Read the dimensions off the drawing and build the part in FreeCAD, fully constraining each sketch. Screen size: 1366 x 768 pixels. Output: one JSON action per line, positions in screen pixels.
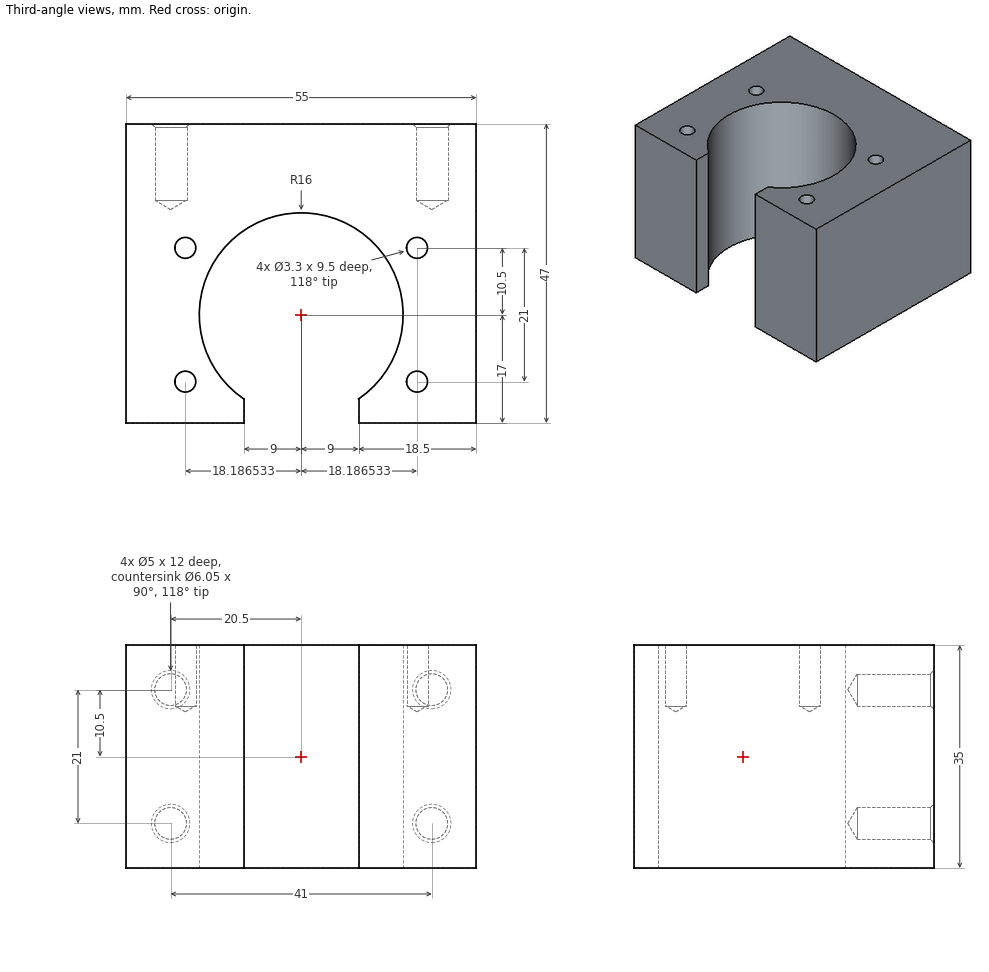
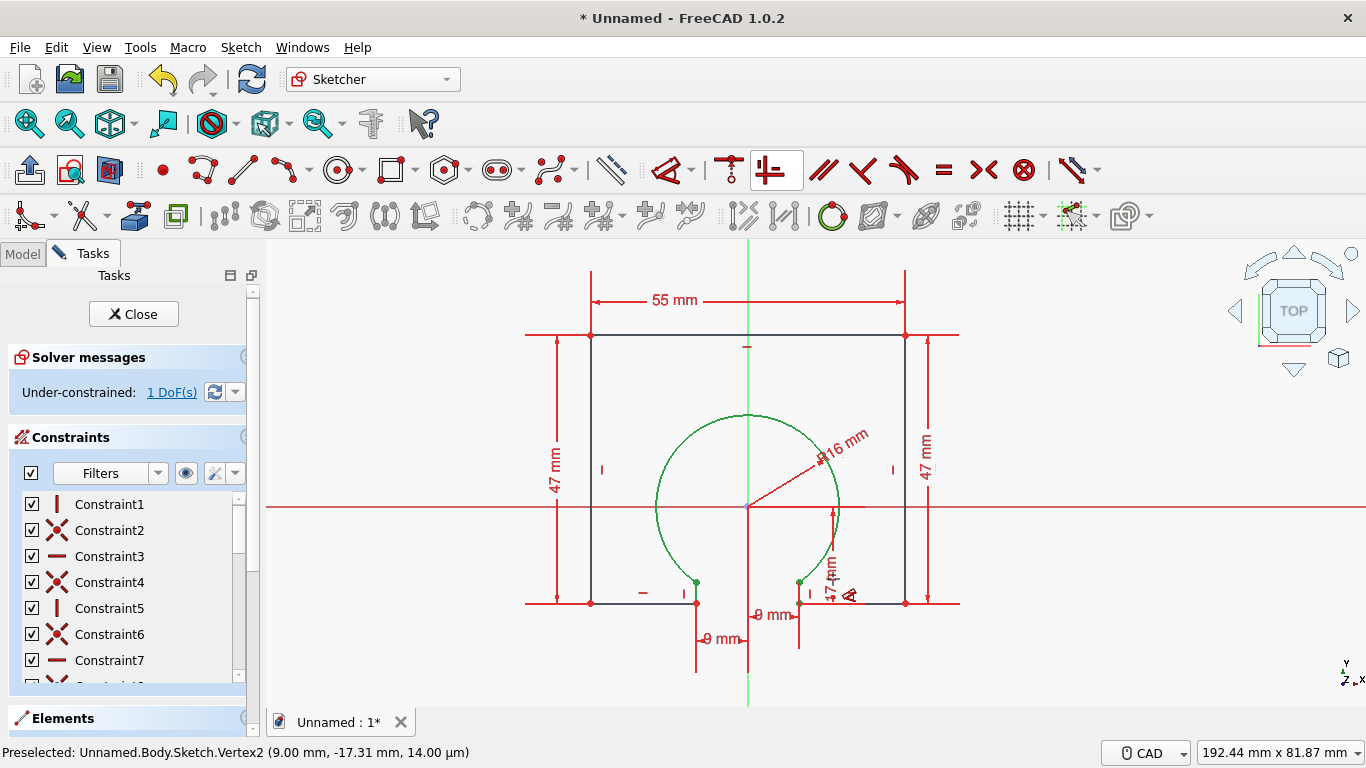
{"action": "left_click", "coordinate": [831, 604]}
{"action": "left_click", "coordinate": [852, 638]}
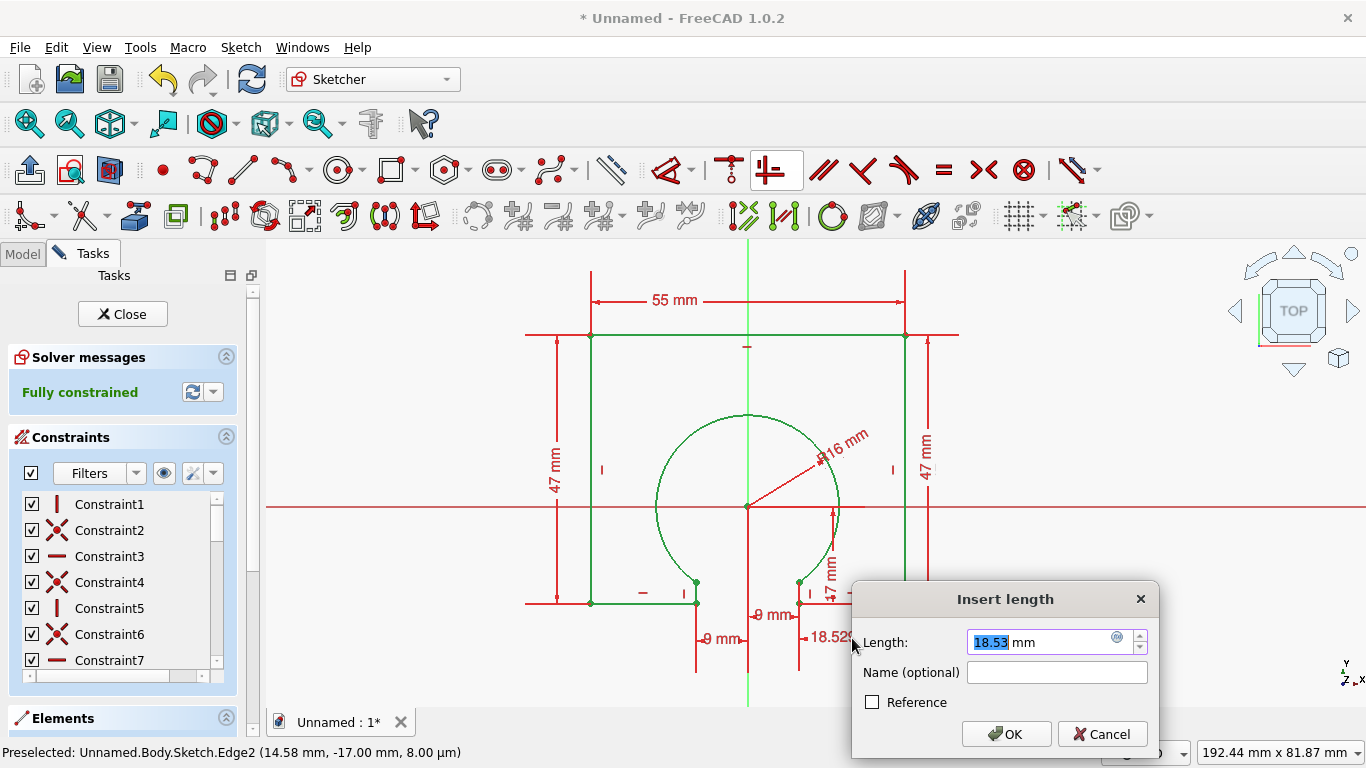
{"action": "type", "text": "18.5"}
{"action": "key", "text": "Return"}
{"action": "key", "text": "Escape"}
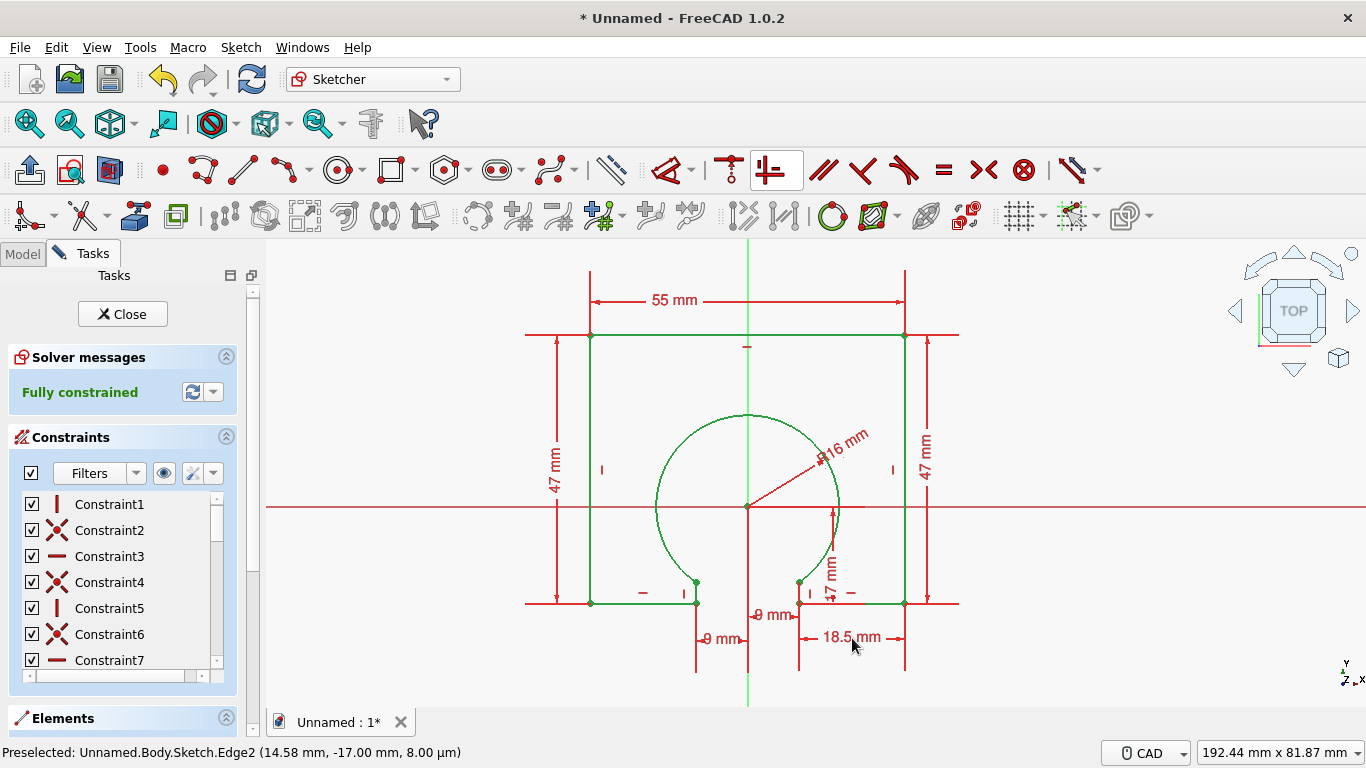
{"action": "left_click", "coordinate": [123, 314]}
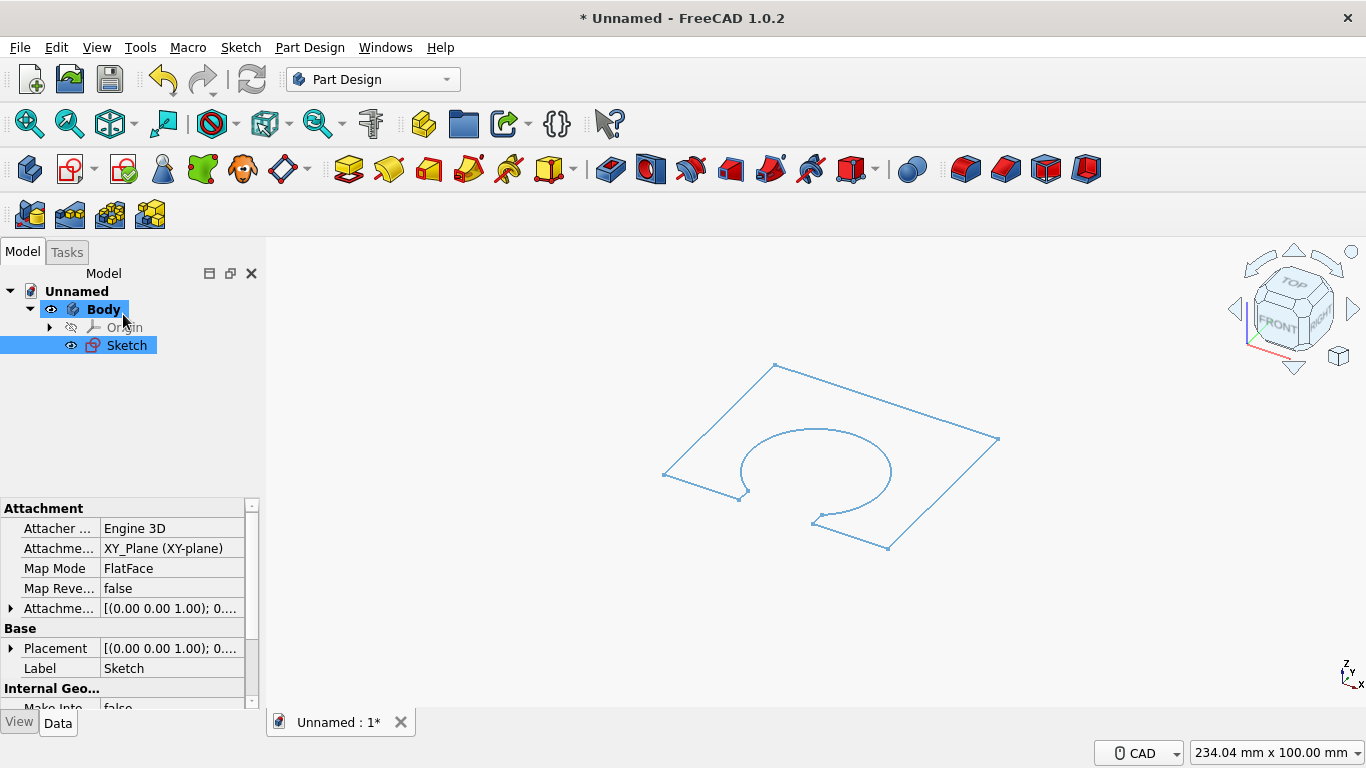
{"action": "left_click", "coordinate": [350, 170]}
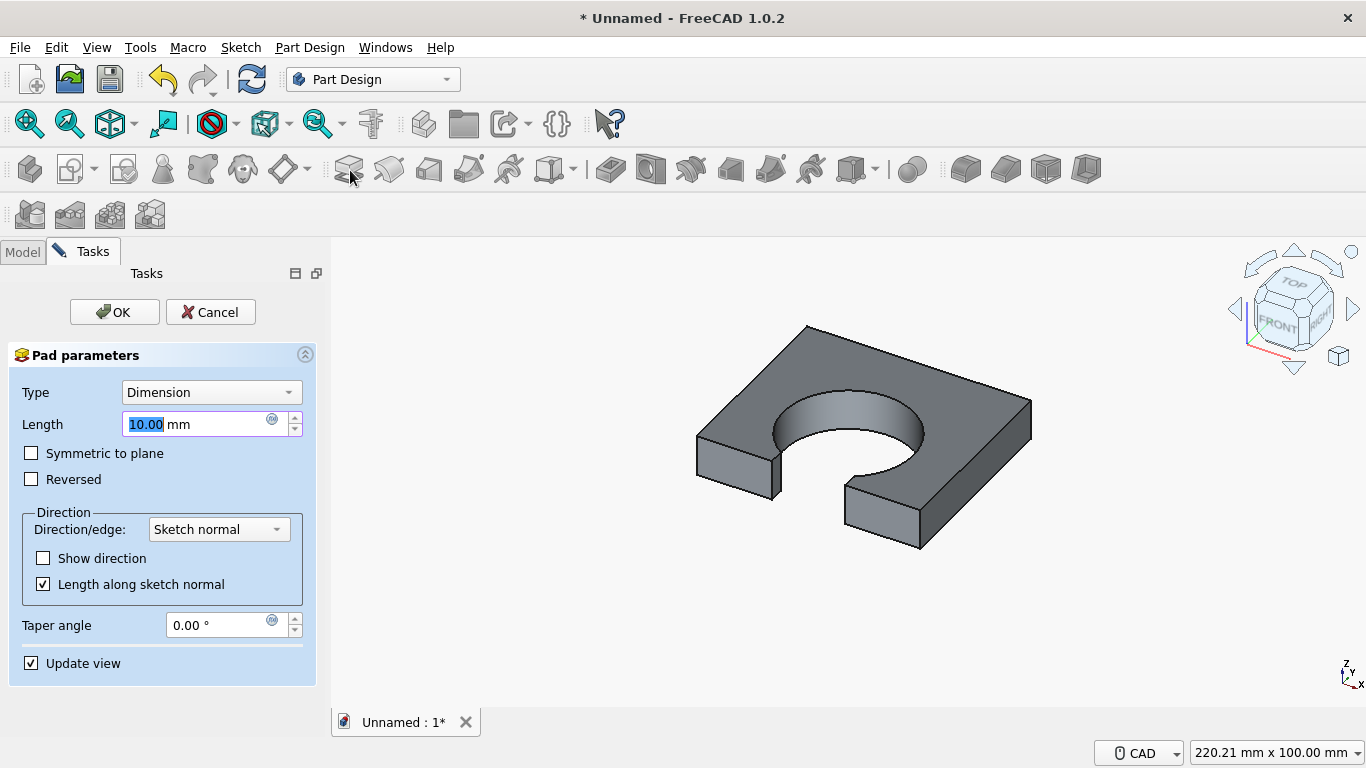
{"action": "type", "text": "35"}
{"action": "key", "text": "Tab"}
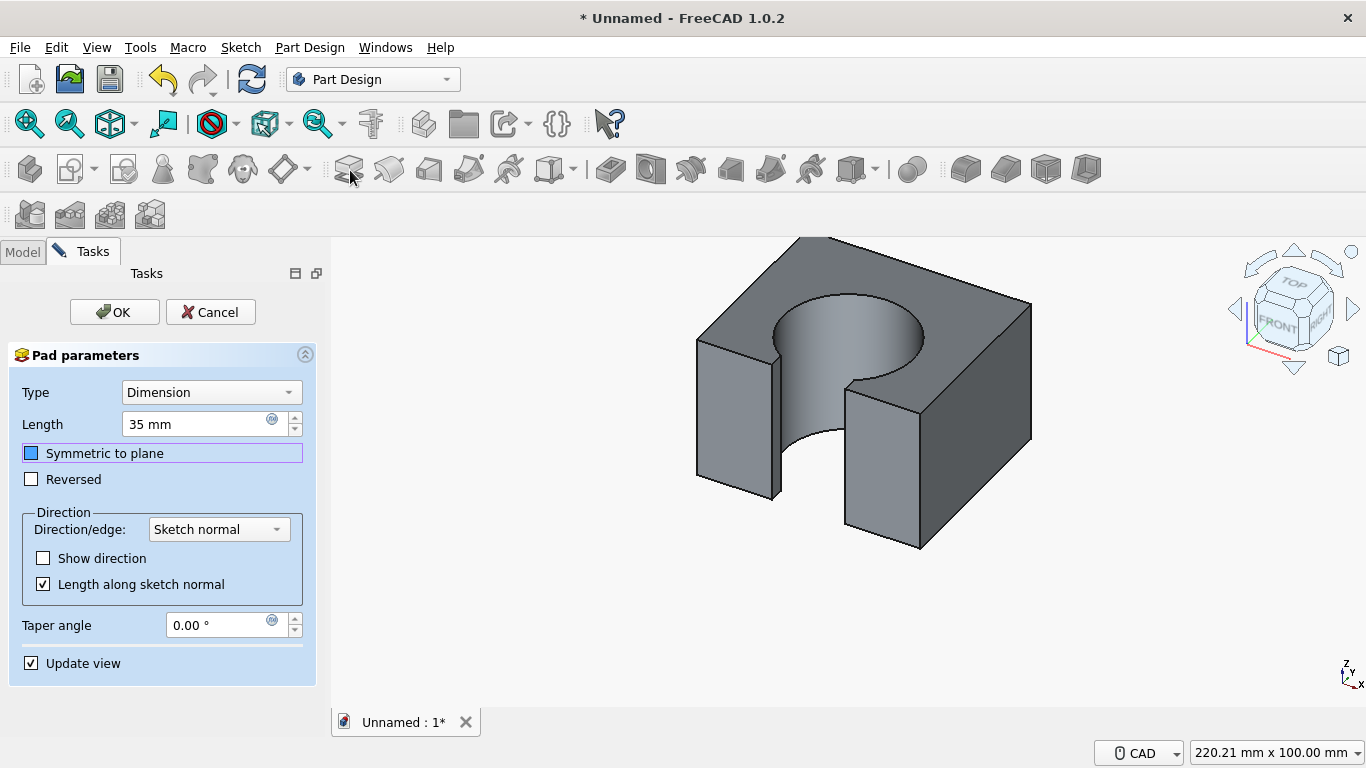
{"action": "left_click", "coordinate": [30, 453]}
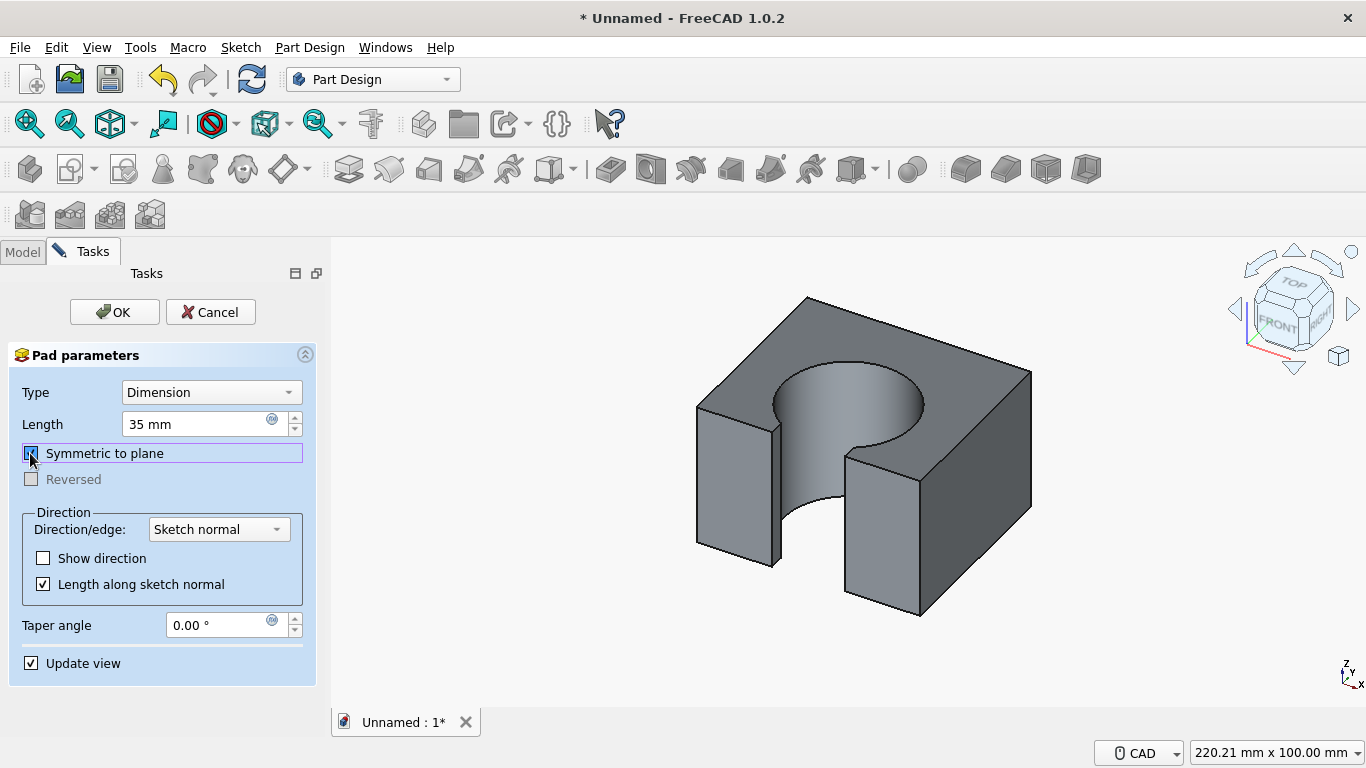
{"action": "left_click", "coordinate": [115, 312]}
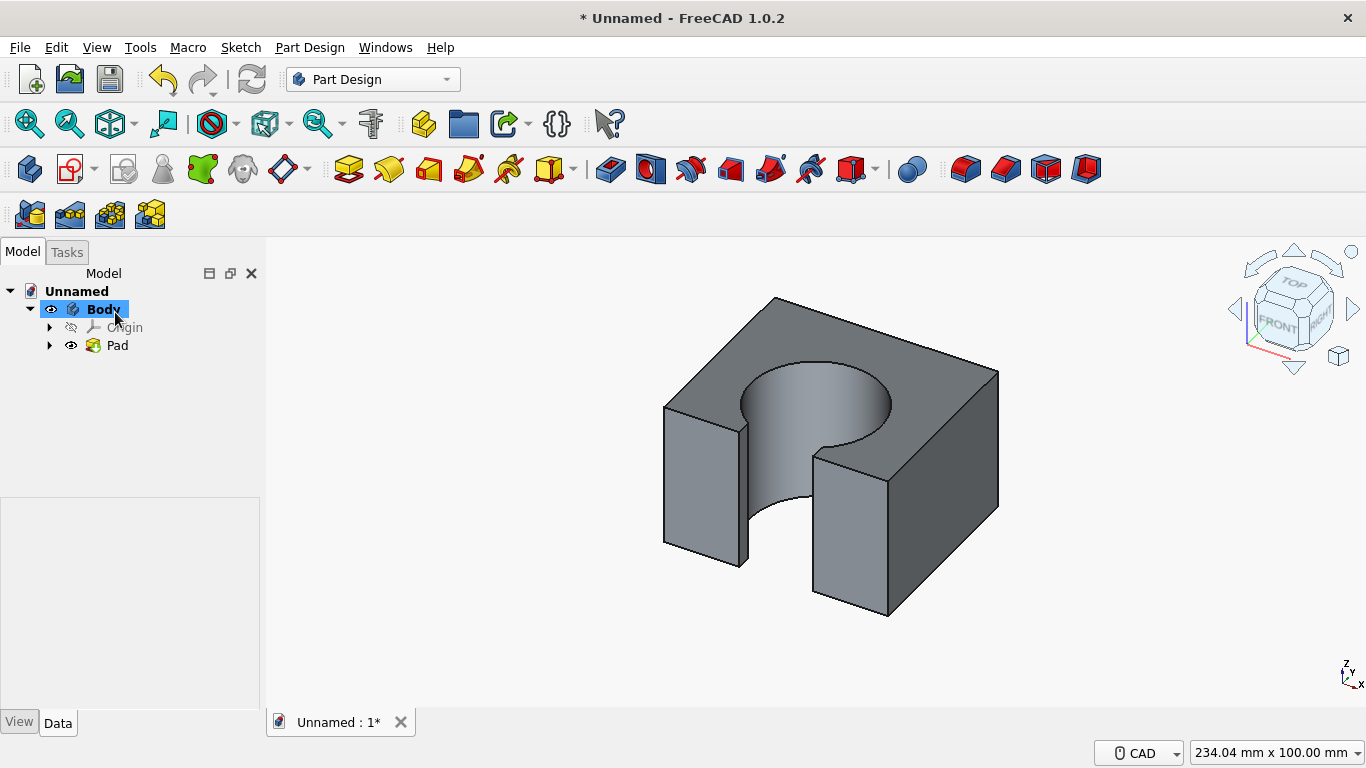
{"action": "left_click", "coordinate": [927, 378]}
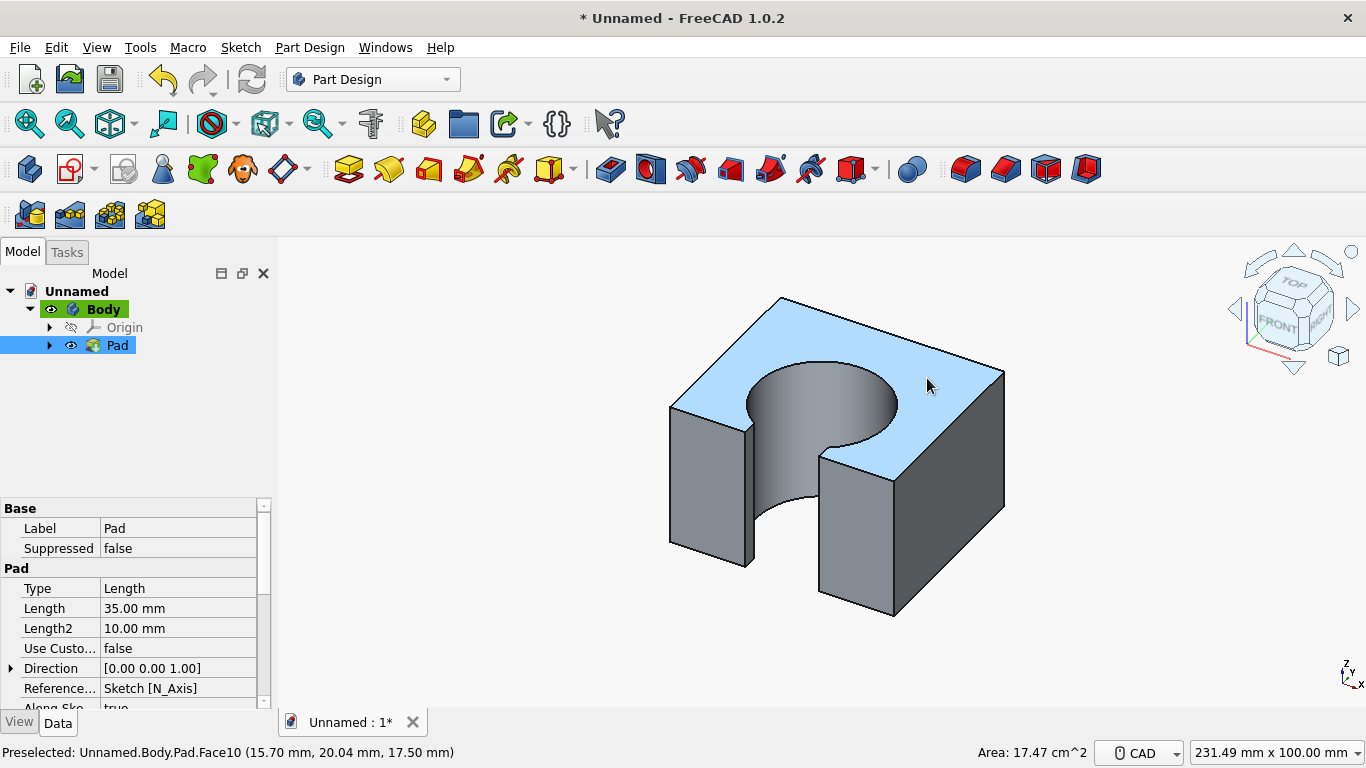
{"action": "left_click", "coordinate": [70, 170]}